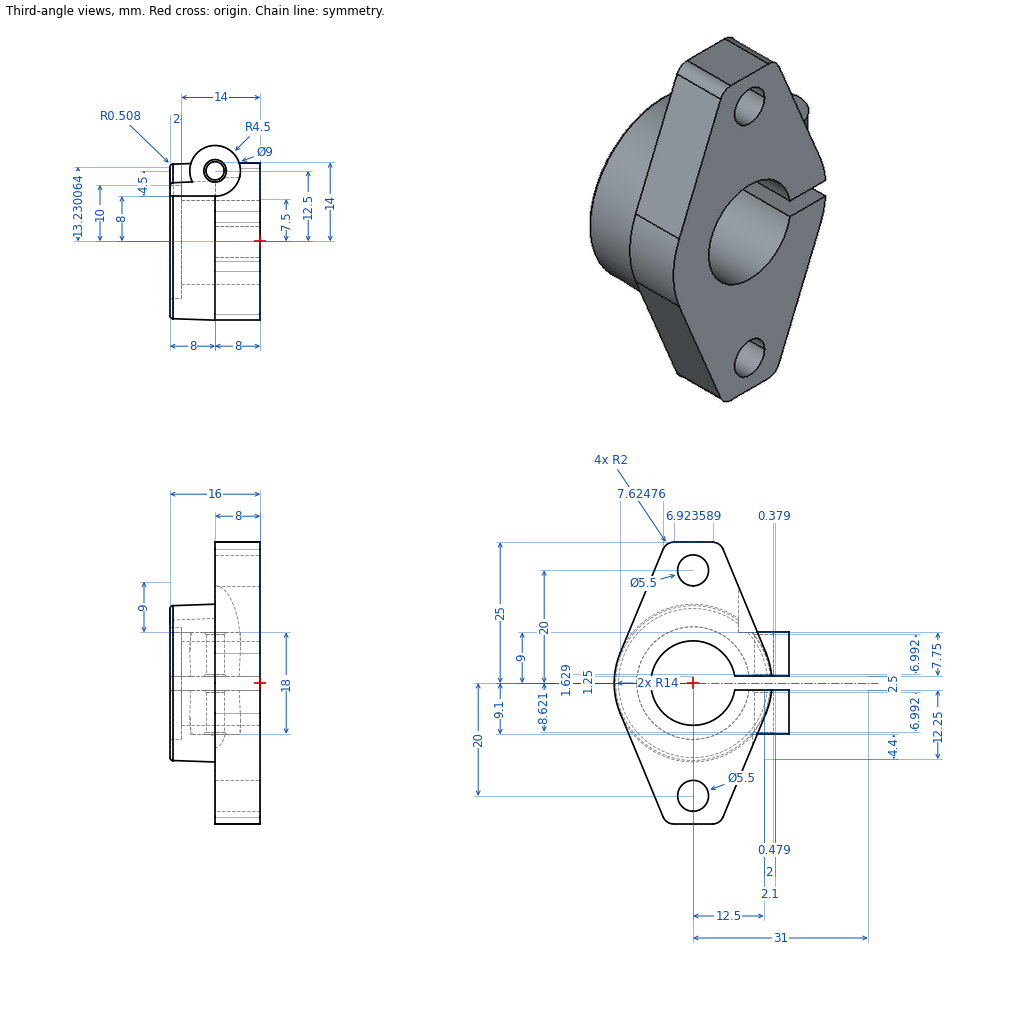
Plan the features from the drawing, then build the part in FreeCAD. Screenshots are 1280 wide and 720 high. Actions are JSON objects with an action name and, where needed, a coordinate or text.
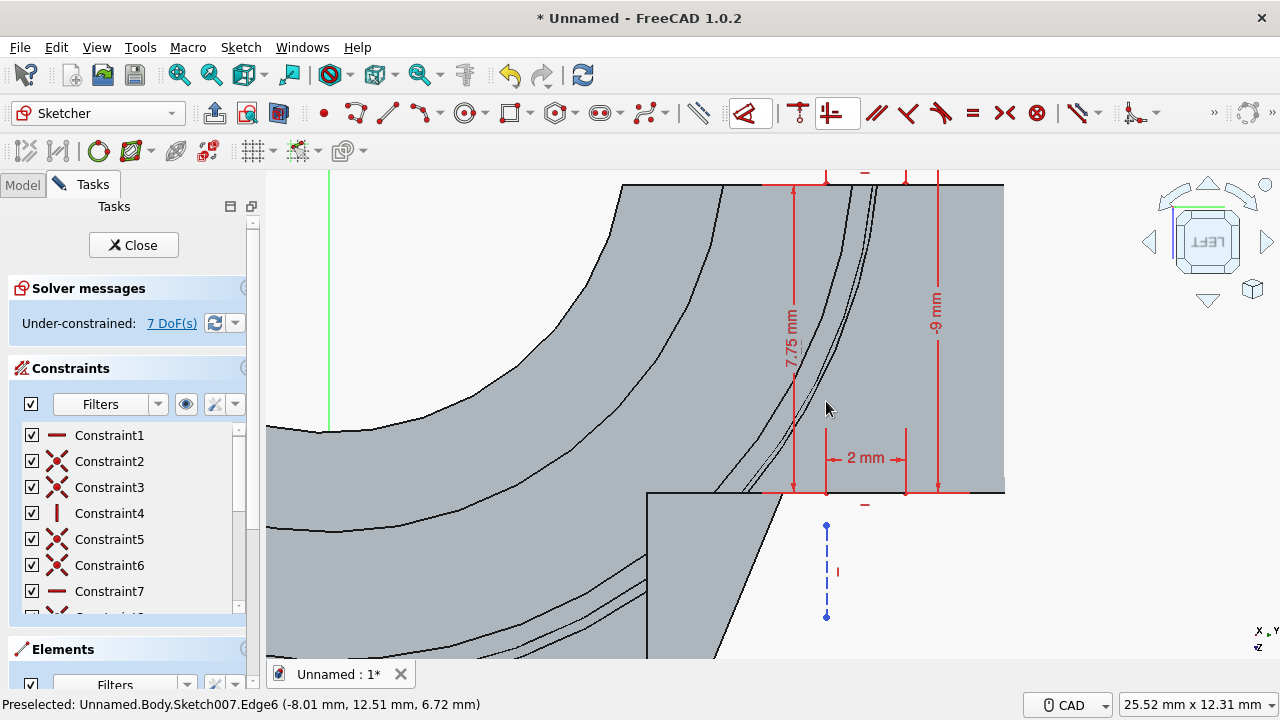
{"action": "left_click", "coordinate": [890, 284]}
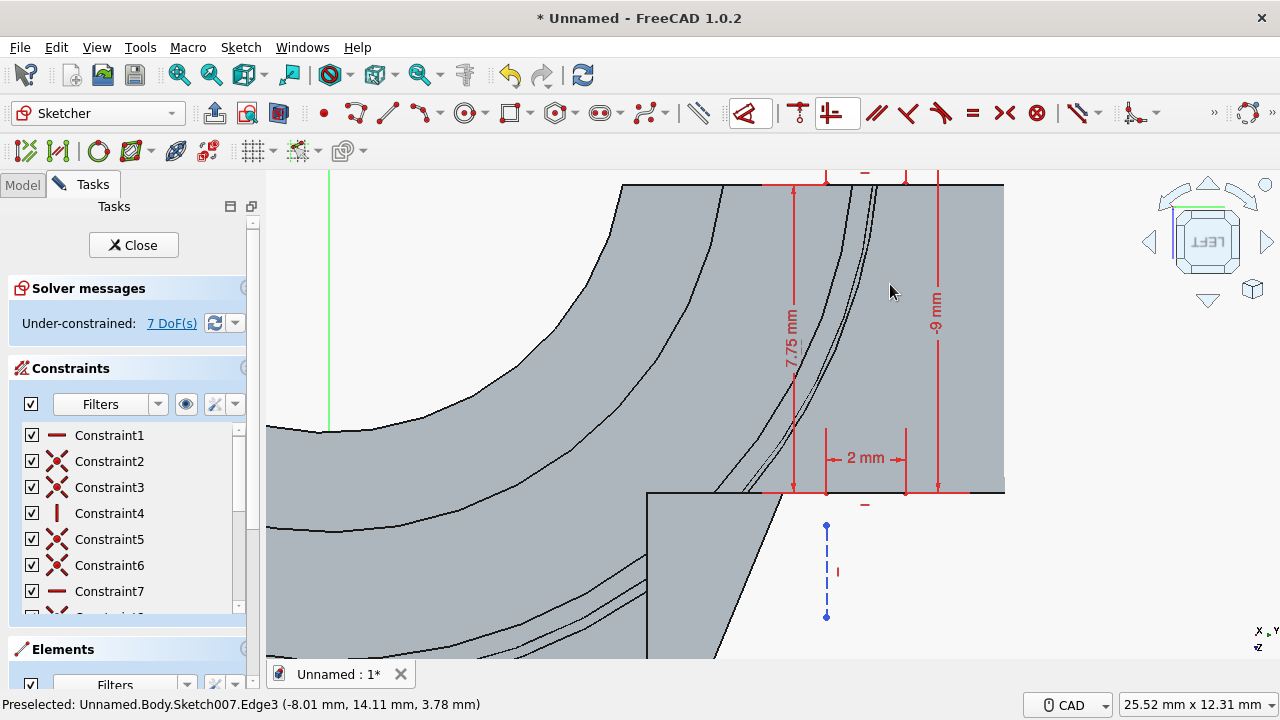
{"action": "left_click", "coordinate": [766, 114]}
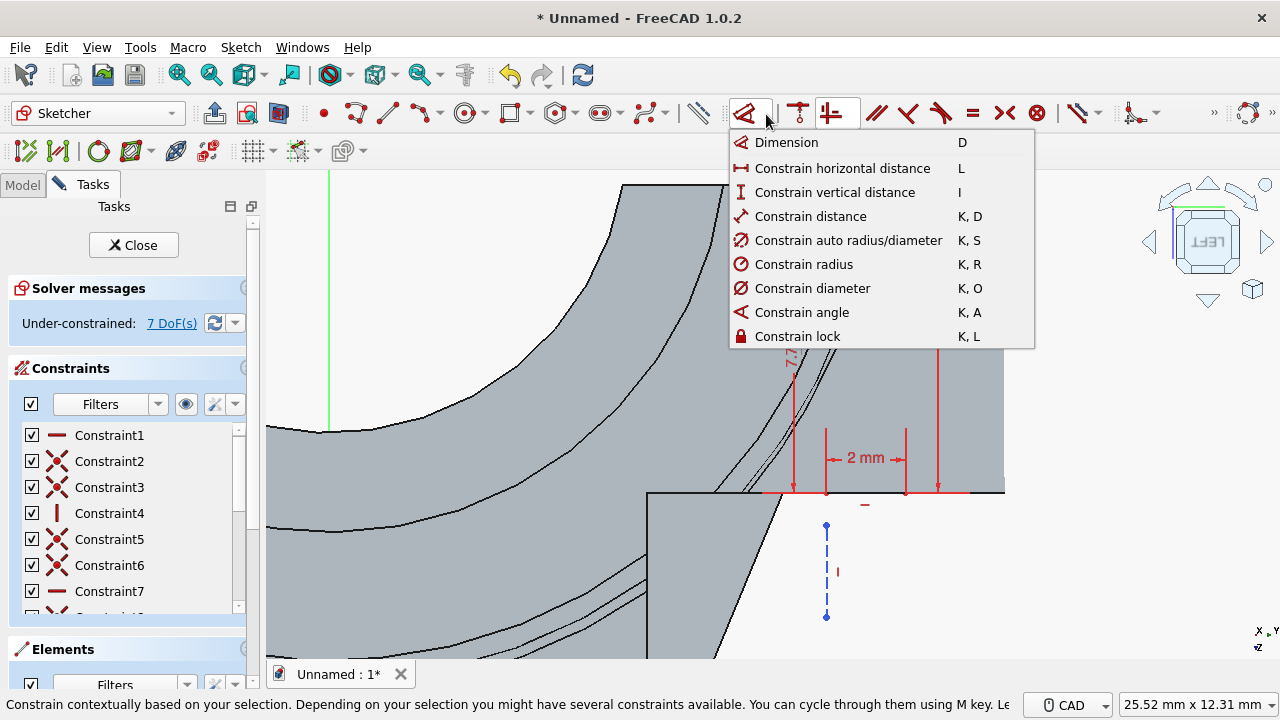
{"action": "left_click", "coordinate": [882, 192]}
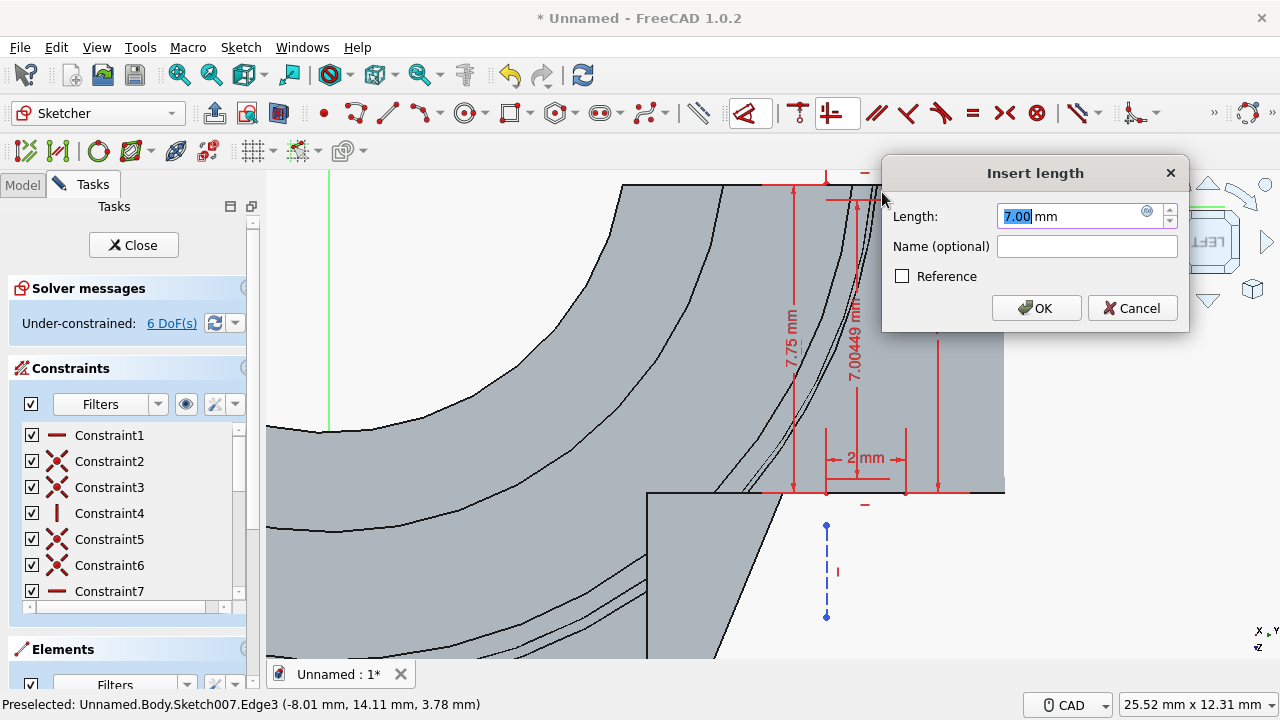
{"action": "type", "text": "6.992"}
{"action": "key", "text": "Return"}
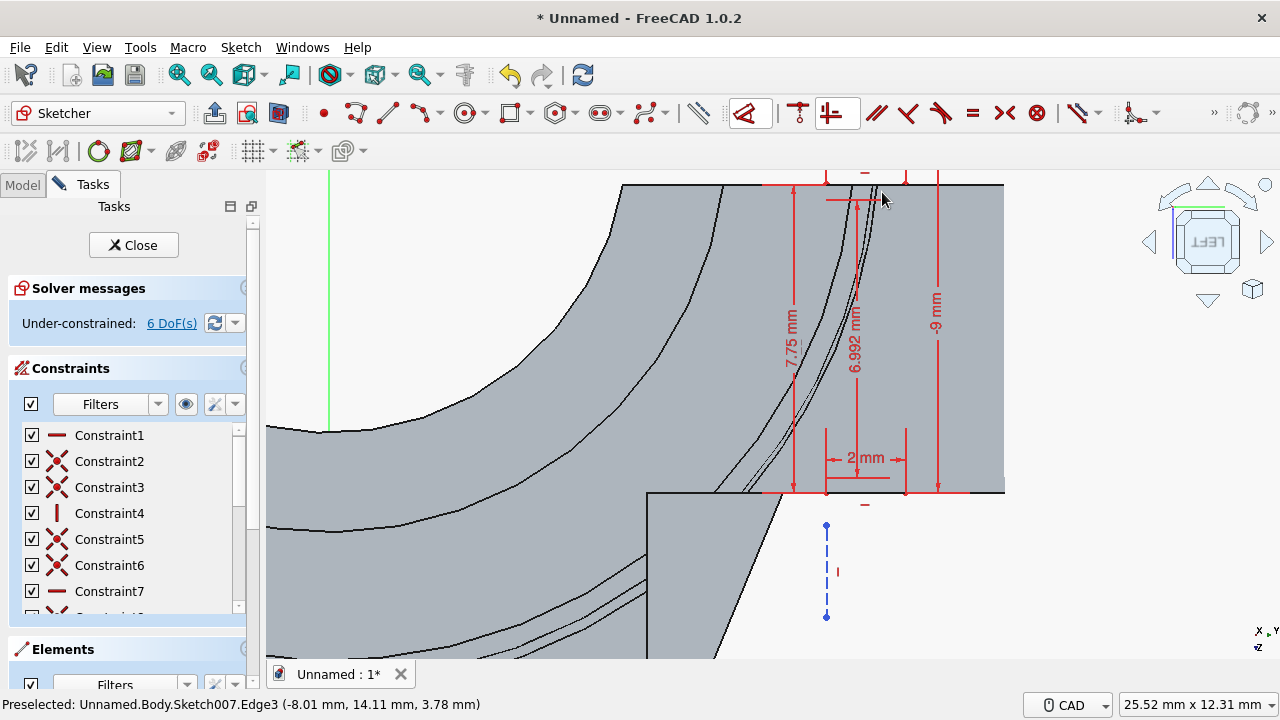
{"action": "scroll", "coordinate": [882, 494], "scroll_direction": "down", "scroll_amount": 2}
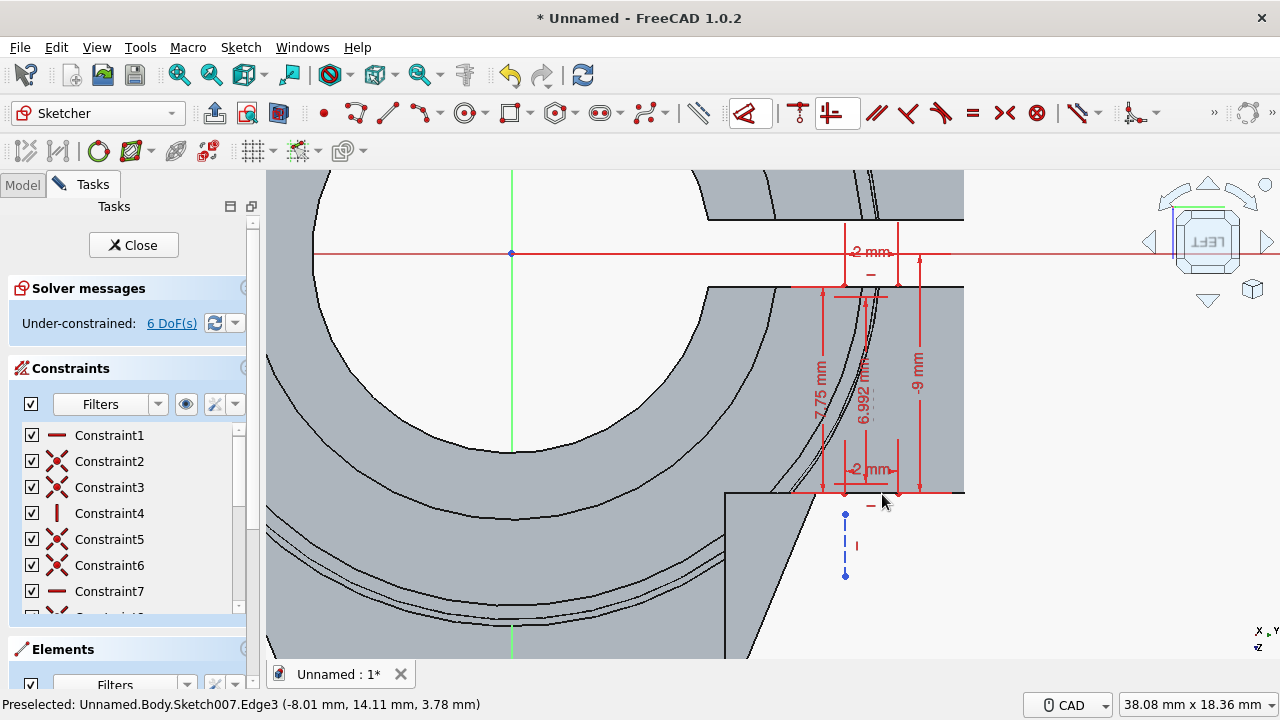
{"action": "left_click", "coordinate": [845, 287]}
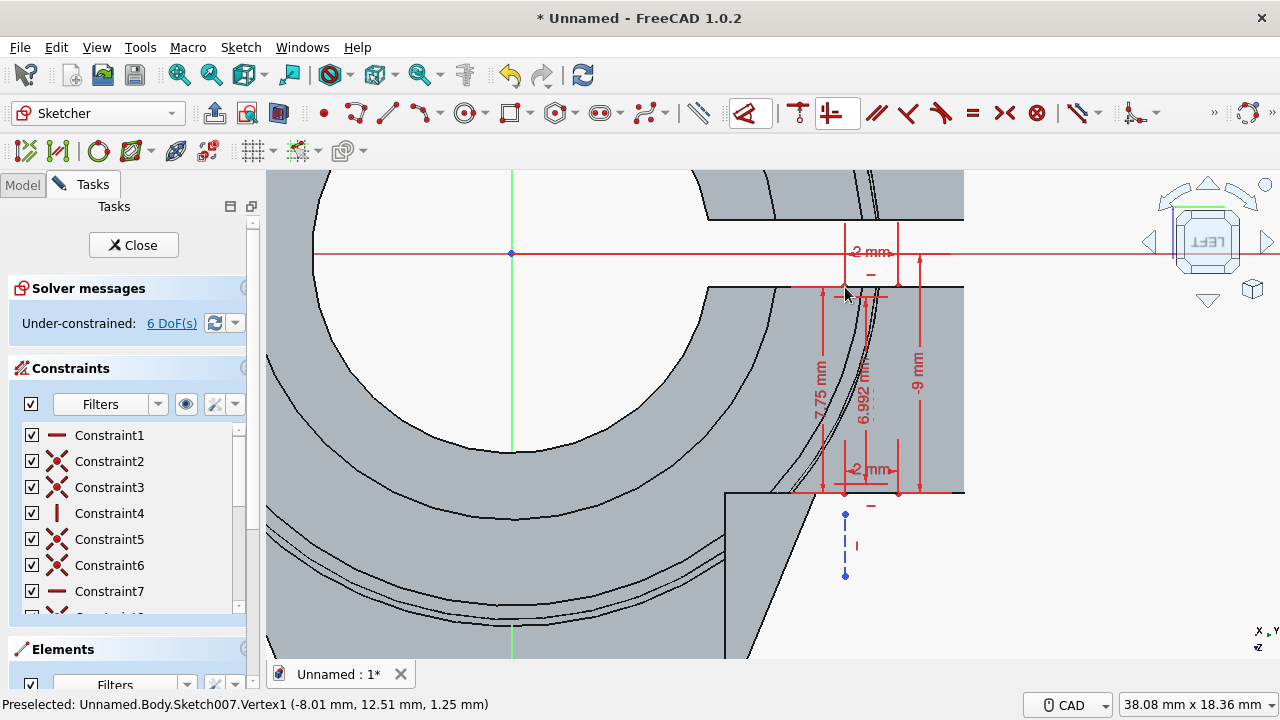
{"action": "left_click", "coordinate": [766, 114]}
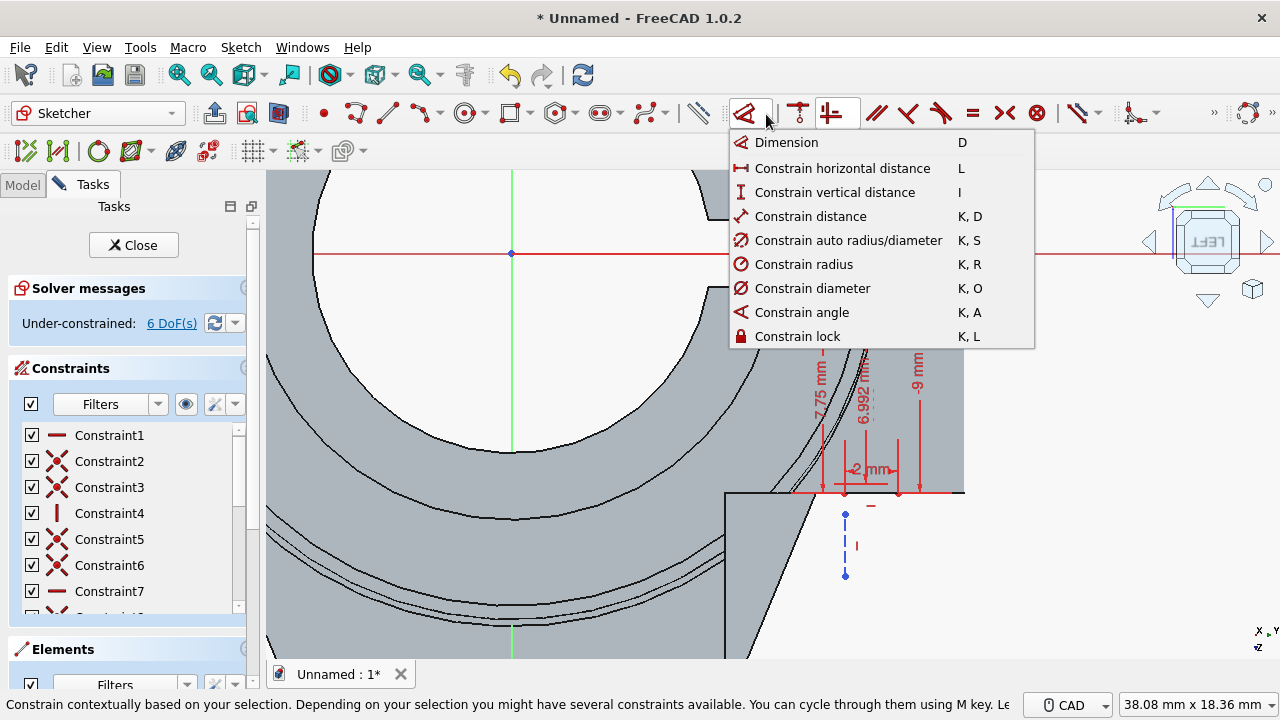
{"action": "left_click", "coordinate": [882, 168]}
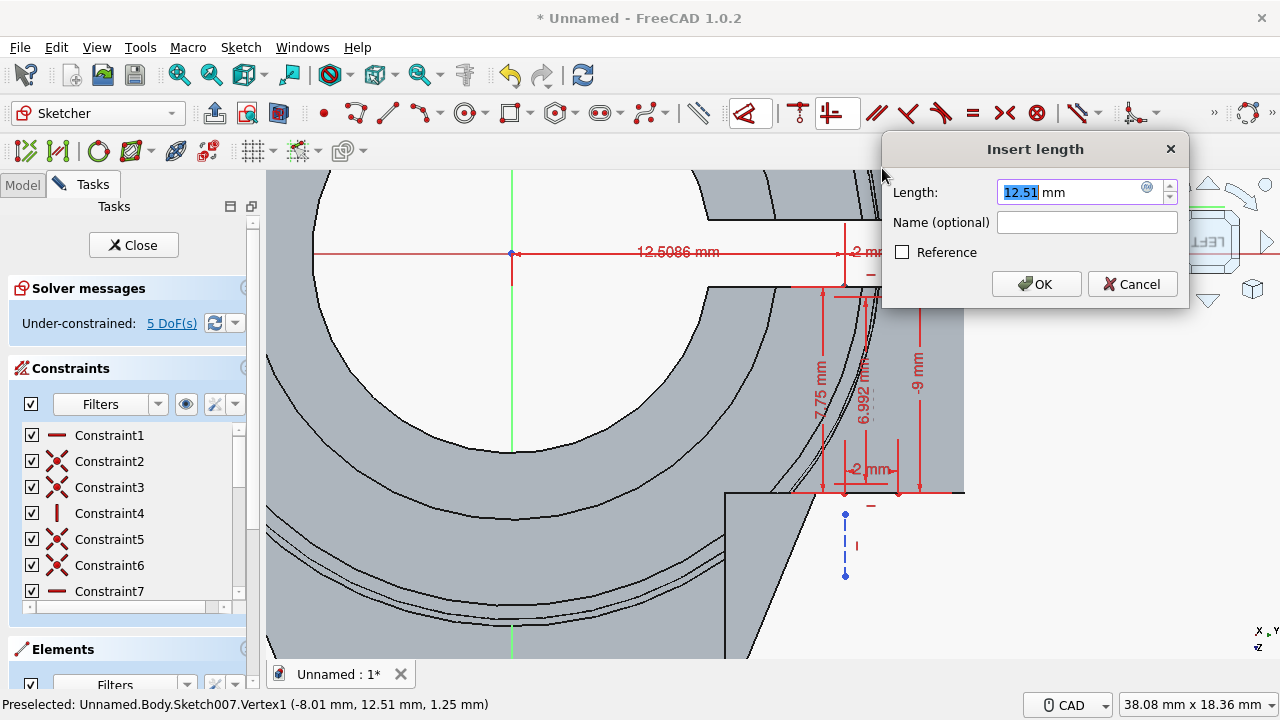
{"action": "type", "text": "12.5"}
{"action": "key", "text": "Return"}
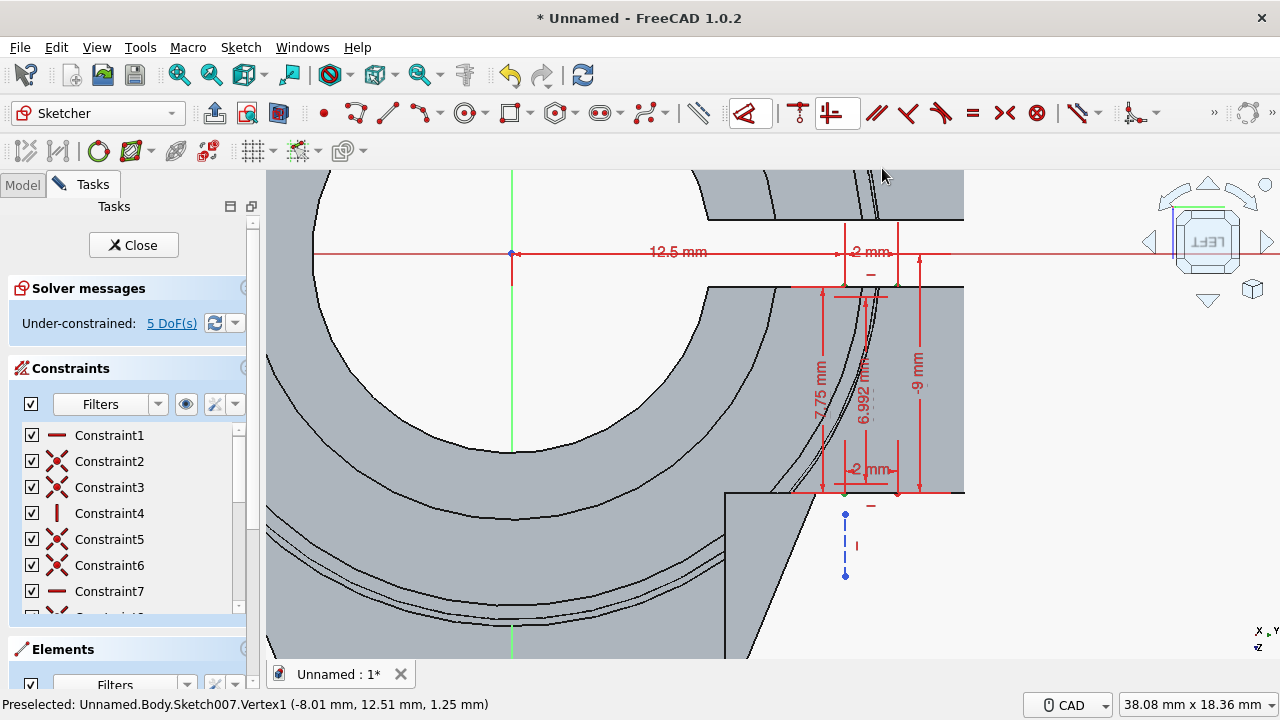
{"action": "left_click", "coordinate": [845, 515]}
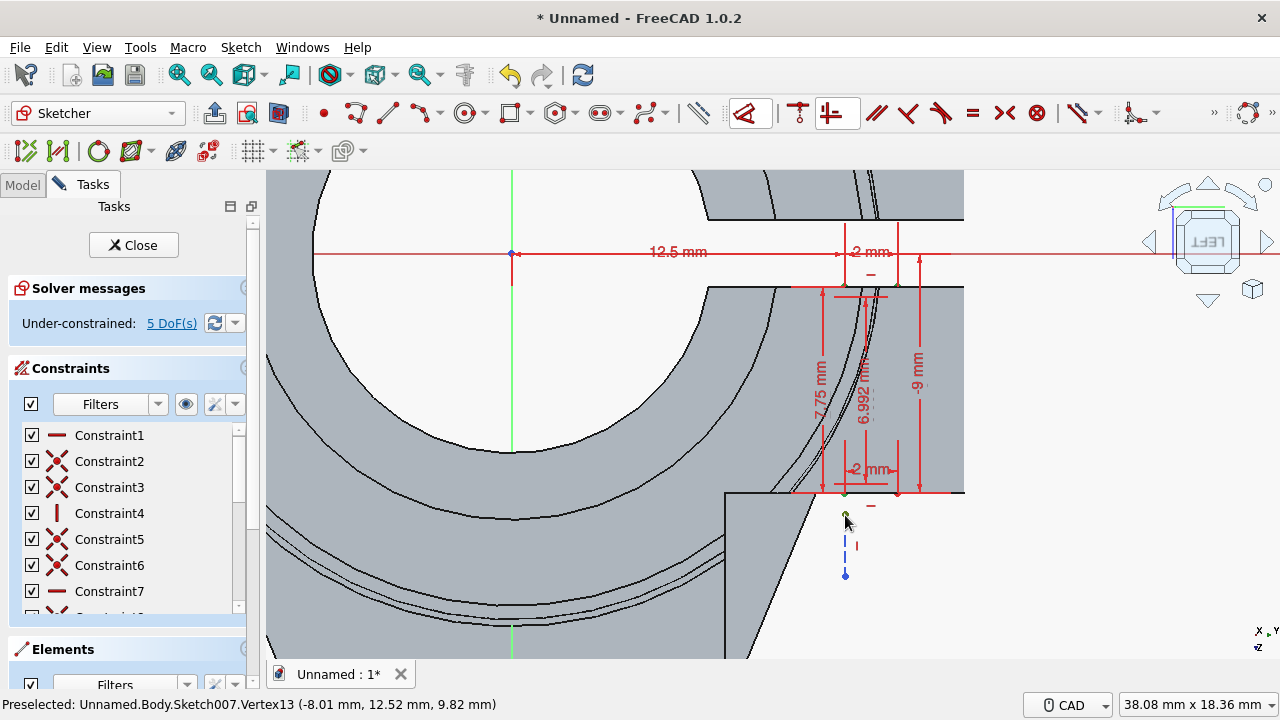
{"action": "left_click", "coordinate": [766, 114]}